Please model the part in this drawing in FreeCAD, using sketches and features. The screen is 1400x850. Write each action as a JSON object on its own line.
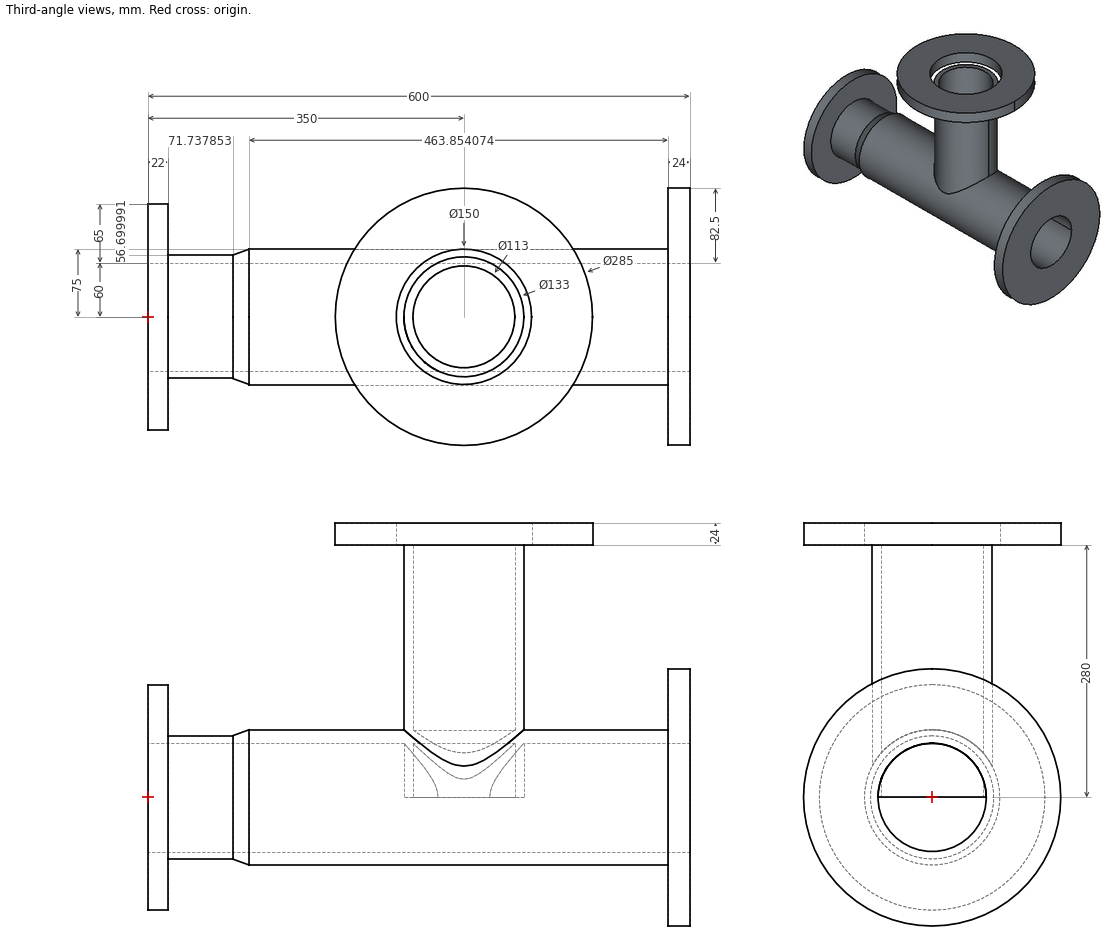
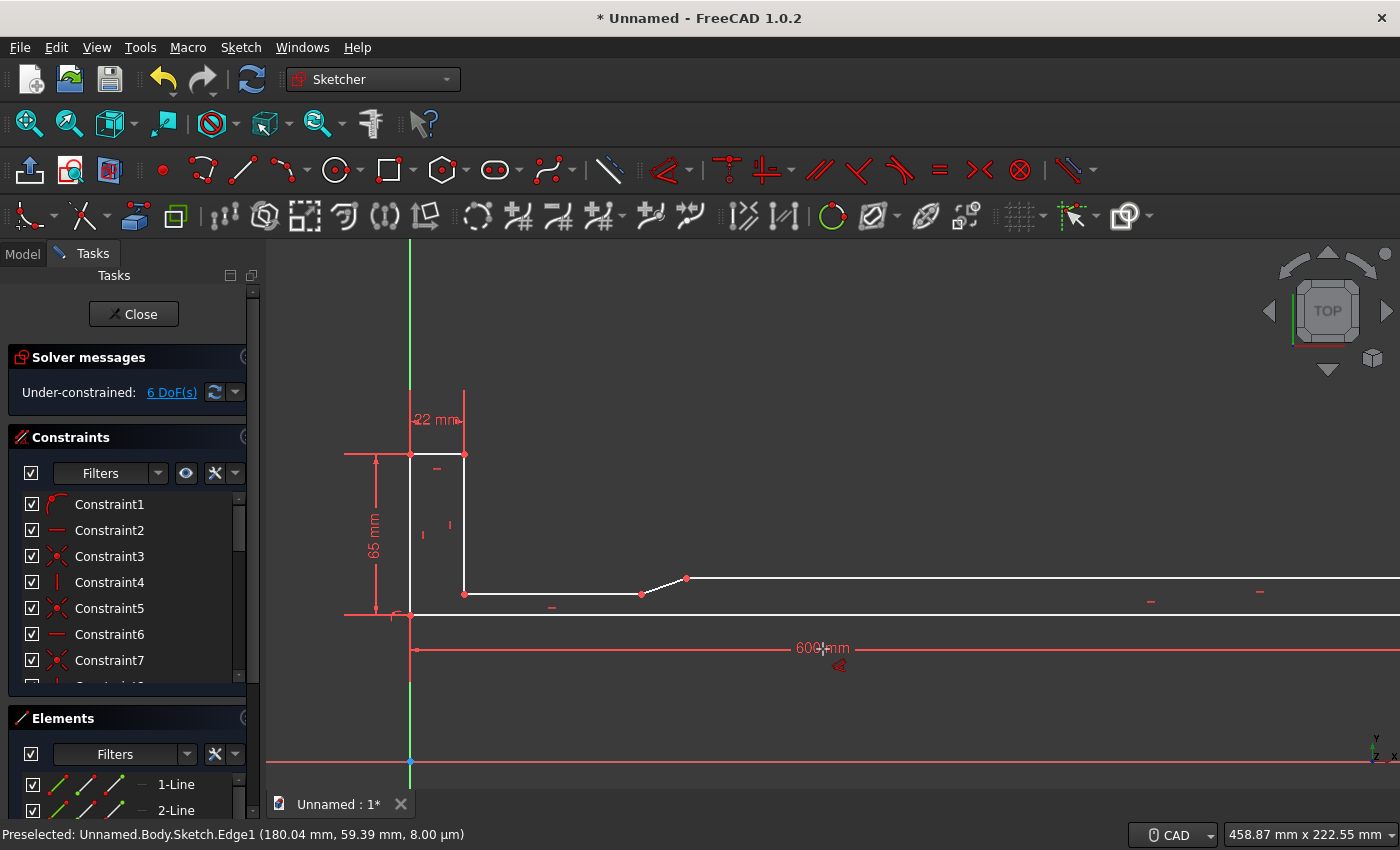
{"action": "left_click", "coordinate": [410, 615]}
{"action": "left_click", "coordinate": [376, 688]}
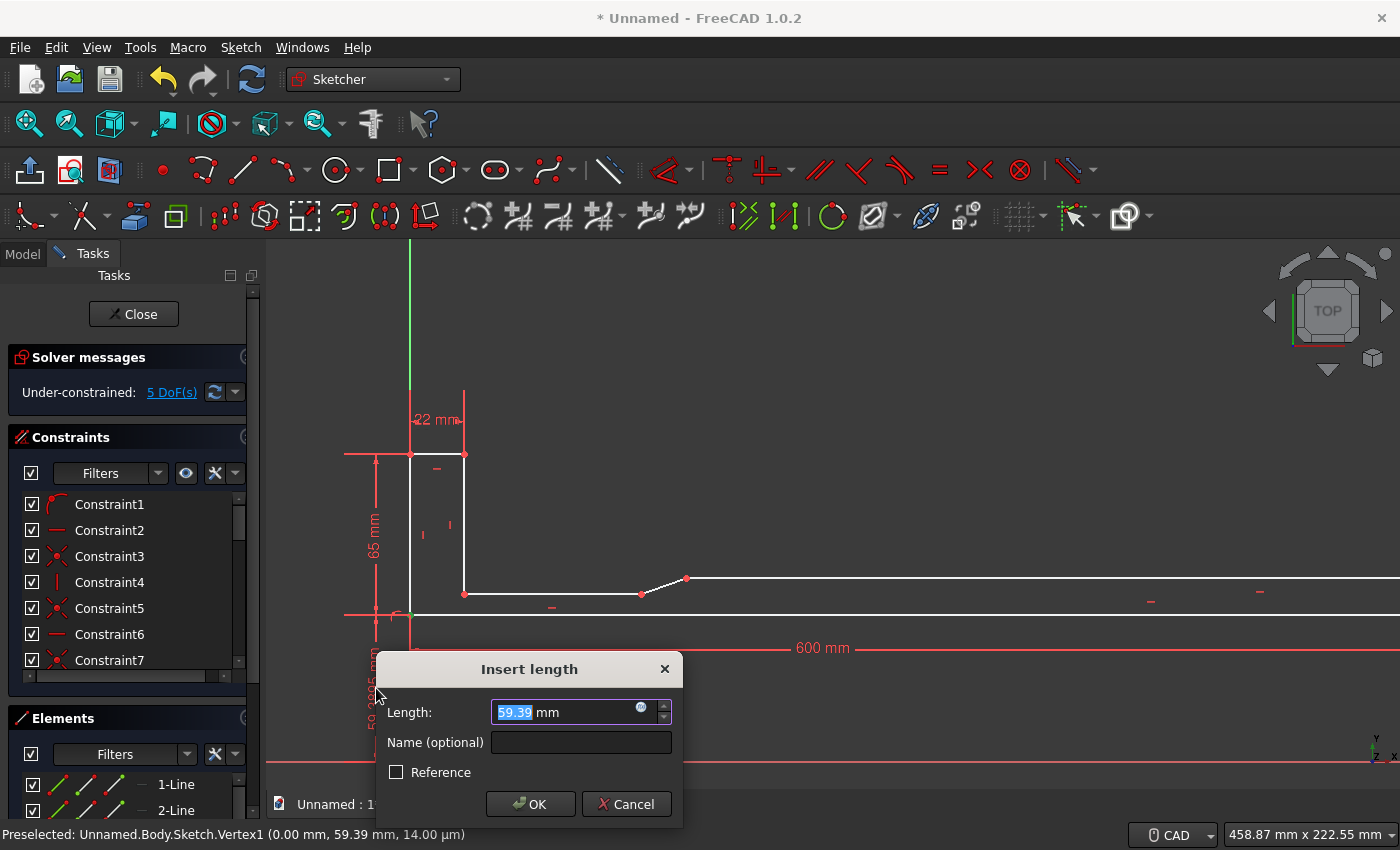
{"action": "type", "text": "60"}
{"action": "key", "text": "Return"}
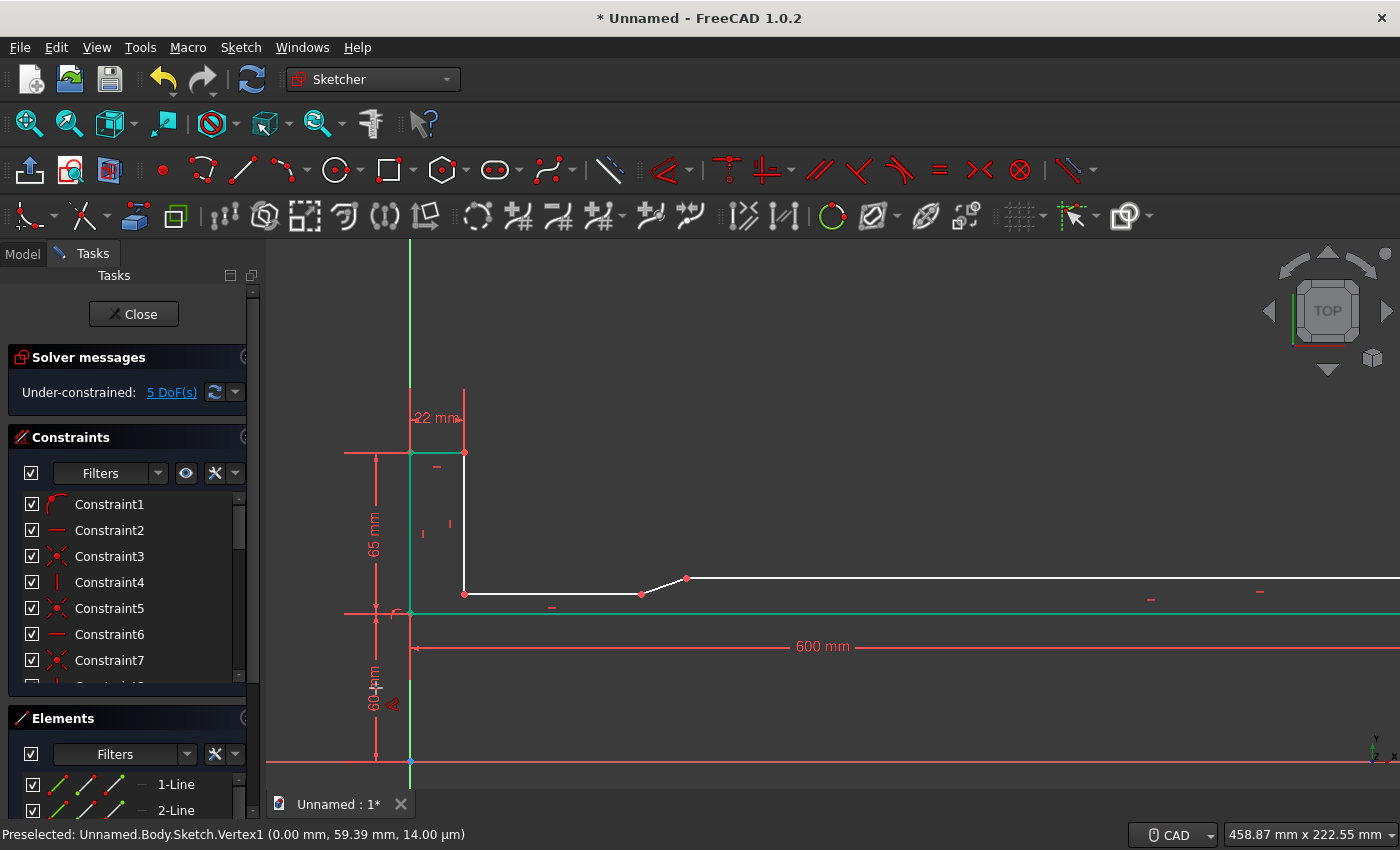
{"action": "scroll", "coordinate": [449, 455], "scroll_direction": "down", "scroll_amount": 4}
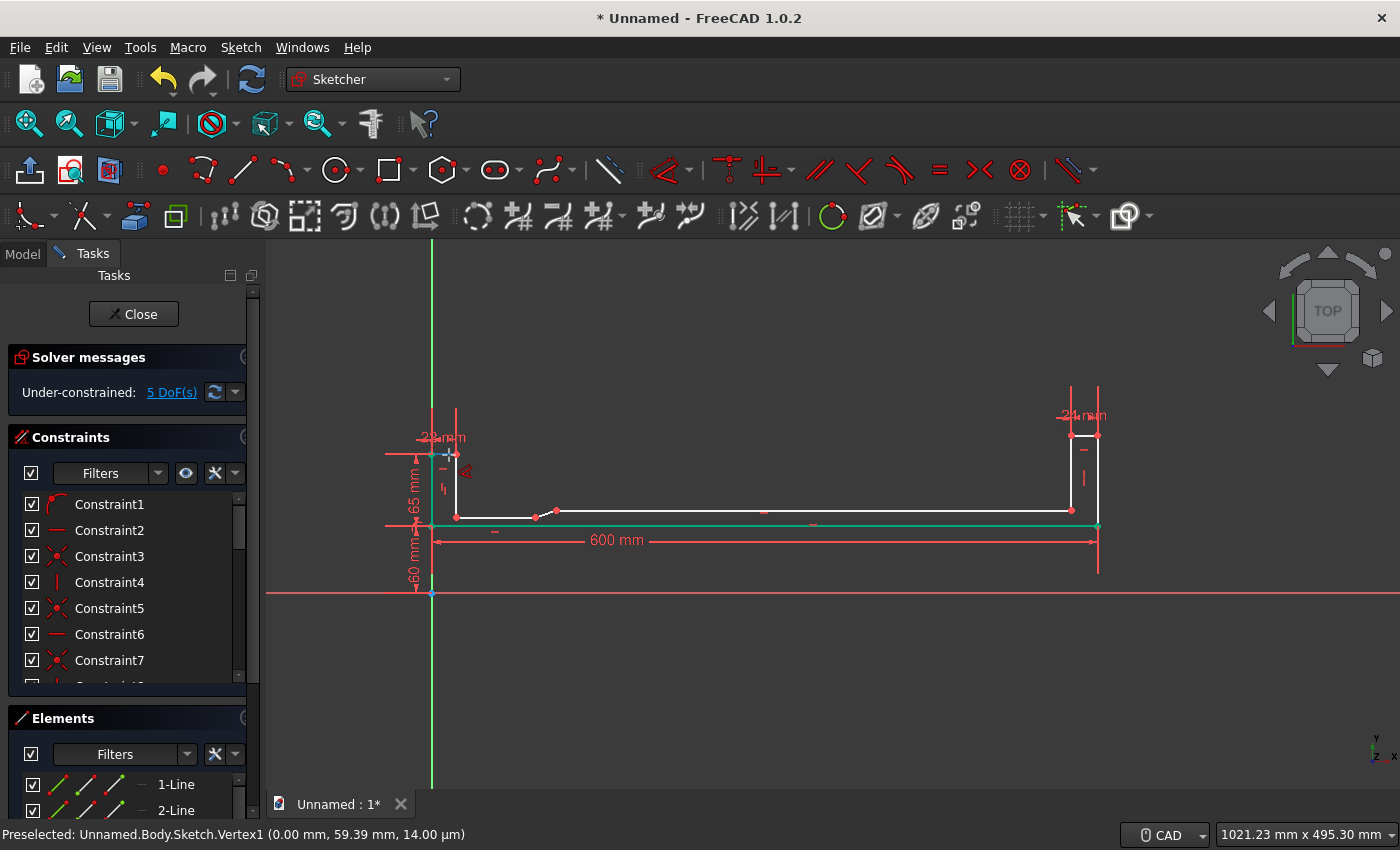
{"action": "left_click", "coordinate": [1071, 511]}
{"action": "left_click", "coordinate": [398, 533]}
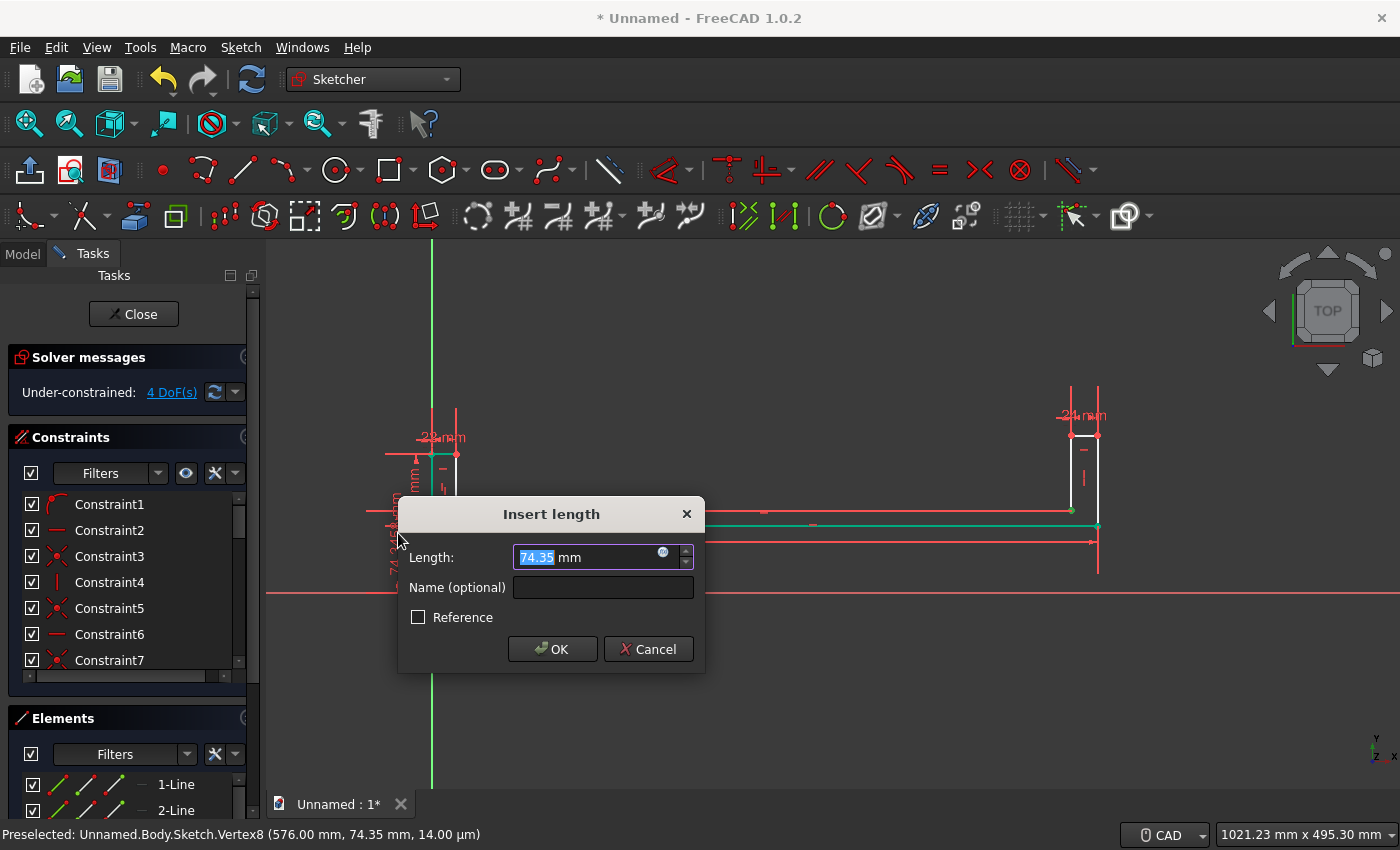
{"action": "type", "text": "75"}
{"action": "key", "text": "Return"}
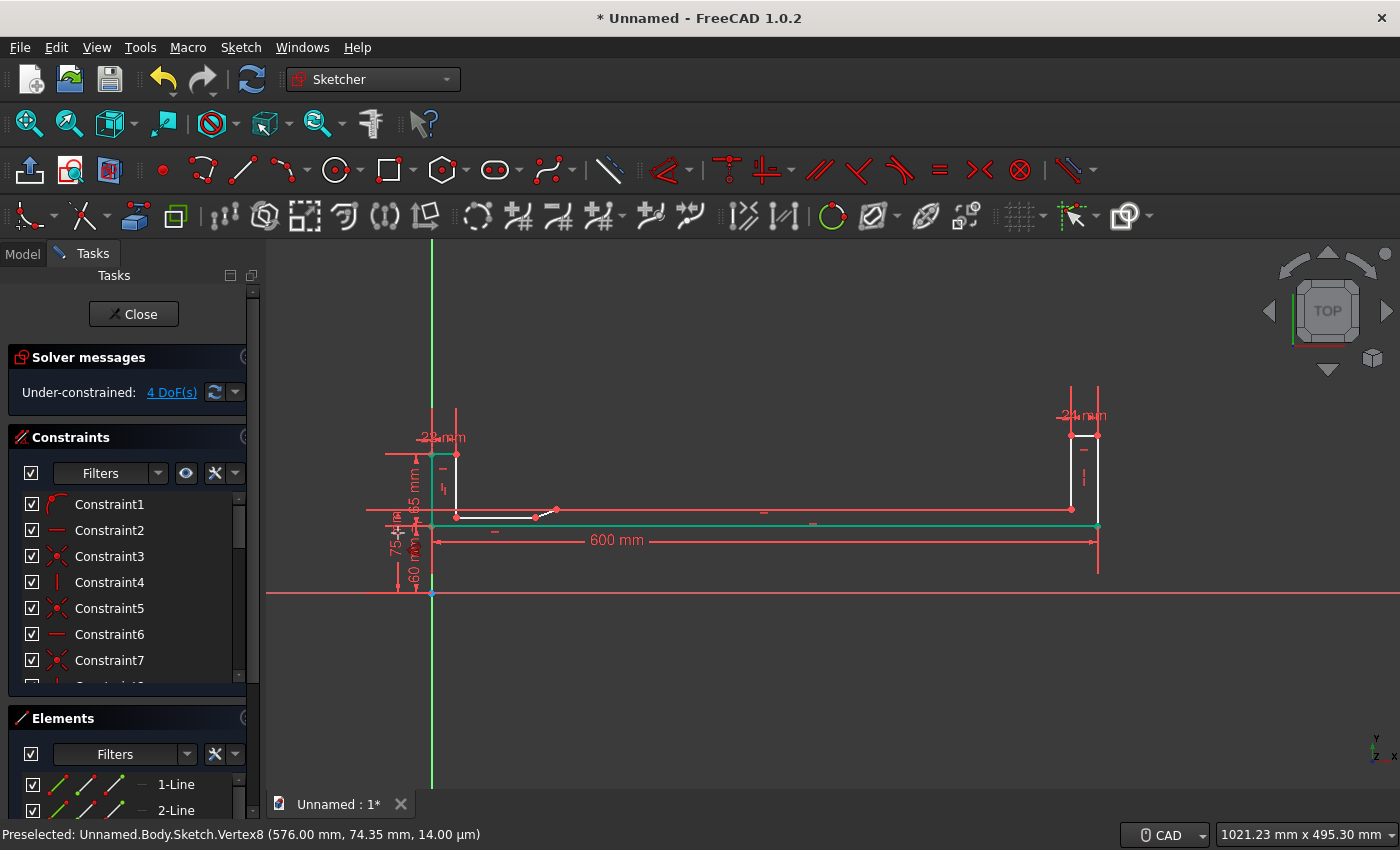
{"action": "left_click", "coordinate": [1098, 499]}
{"action": "left_click", "coordinate": [1132, 481]}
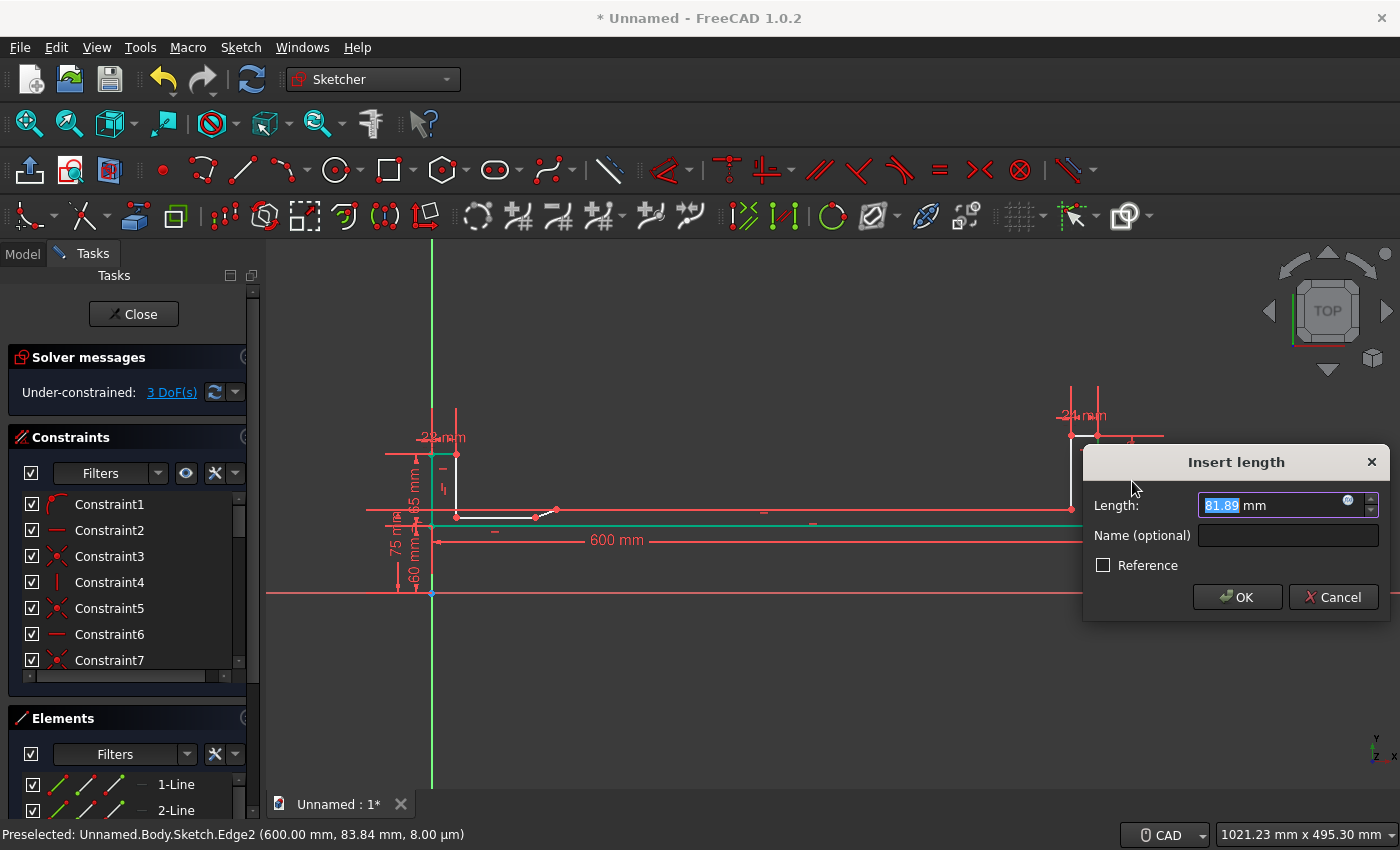
{"action": "type", "text": "82.5"}
{"action": "key", "text": "Return"}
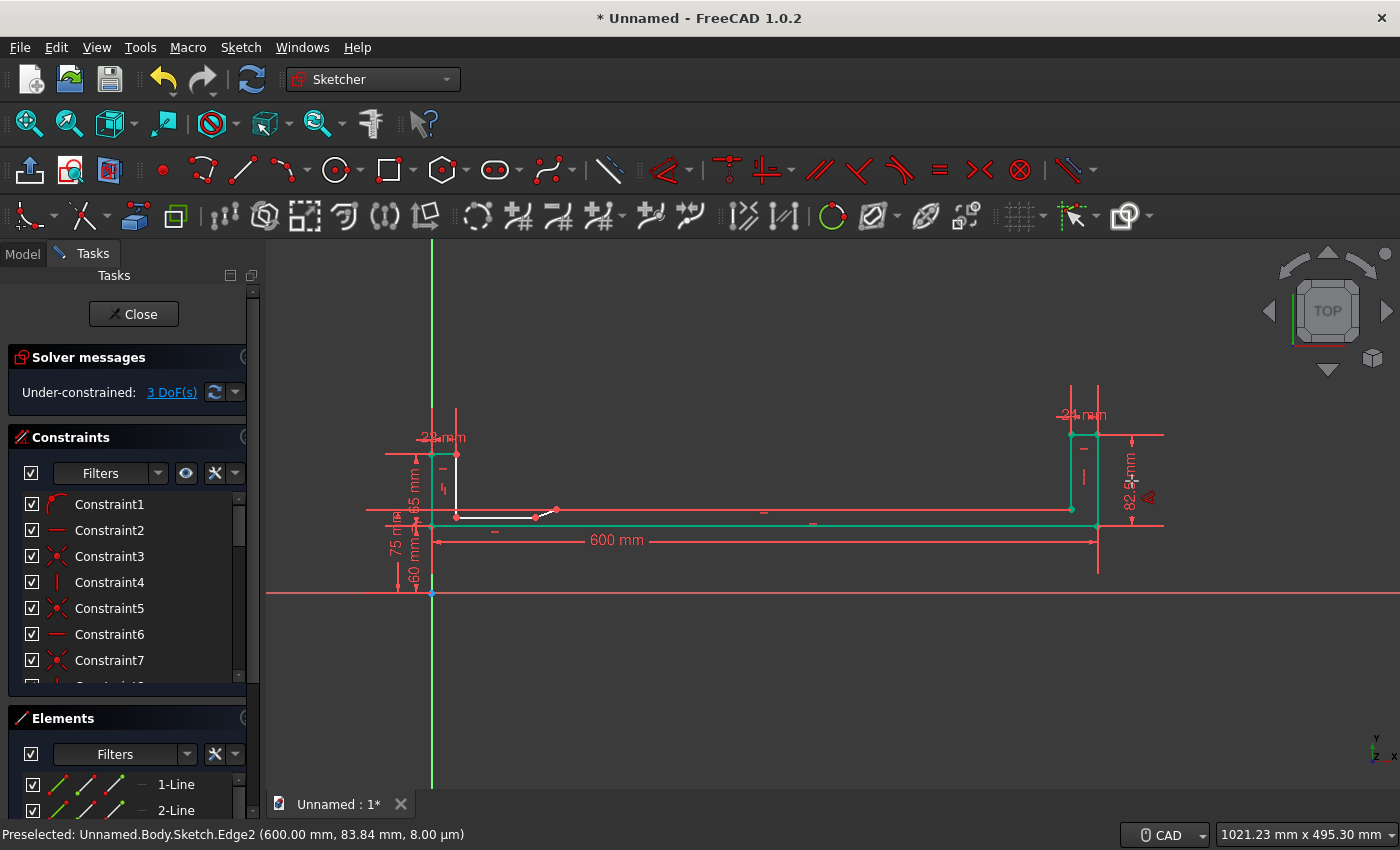
{"action": "scroll", "coordinate": [512, 518], "scroll_direction": "up", "scroll_amount": 3}